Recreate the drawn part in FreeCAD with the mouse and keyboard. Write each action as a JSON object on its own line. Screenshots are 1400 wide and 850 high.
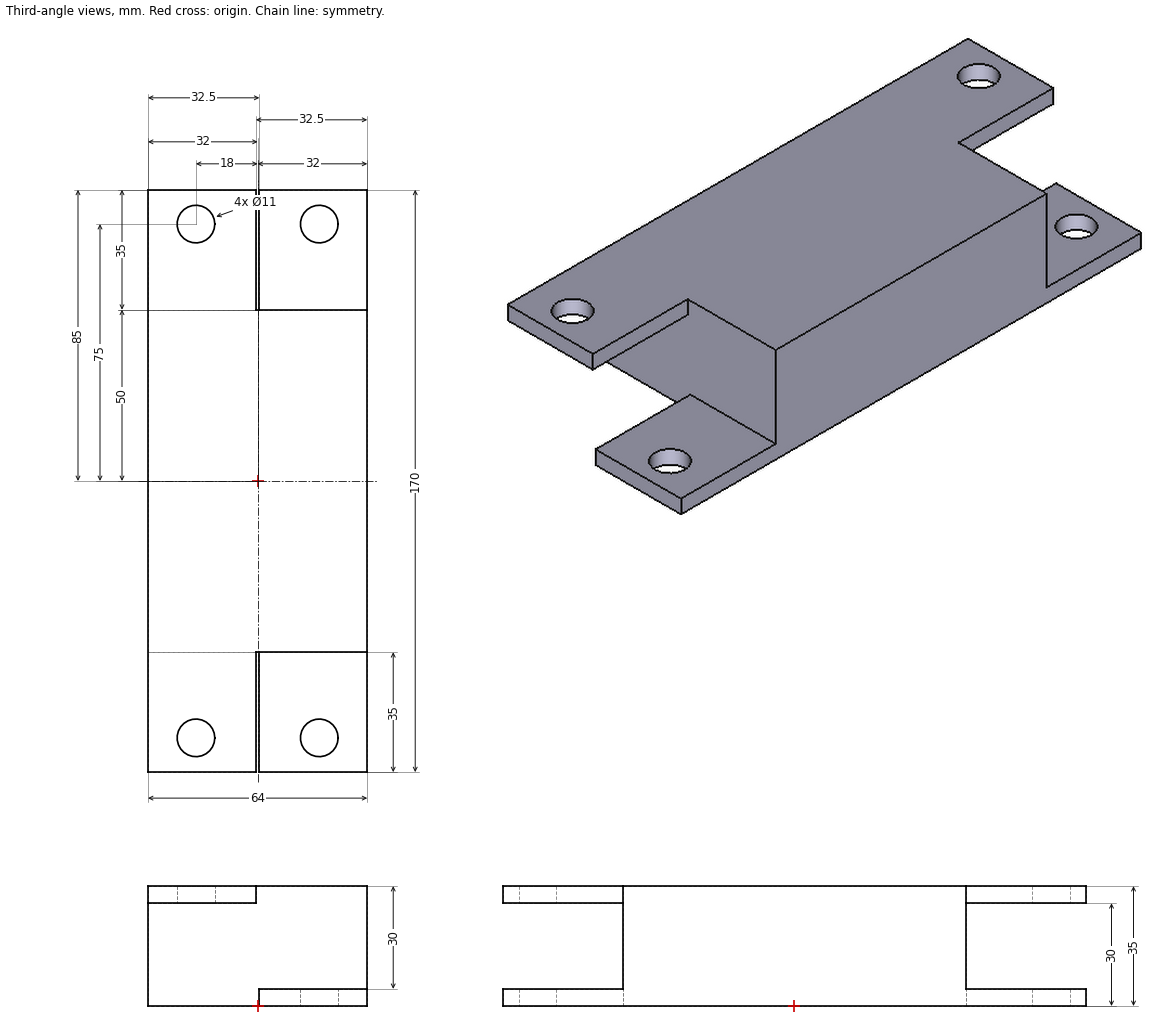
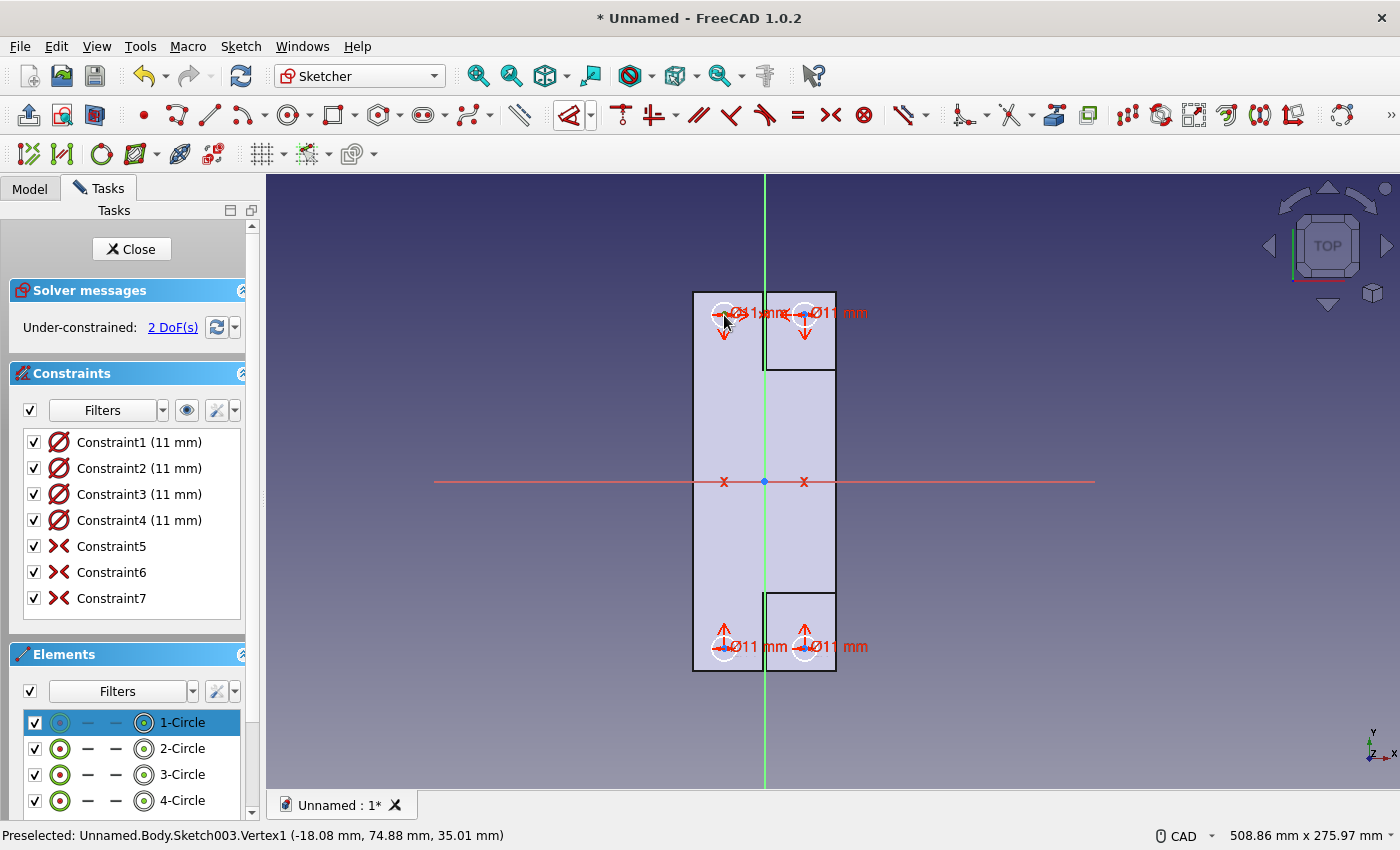
{"action": "left_click", "coordinate": [590, 116]}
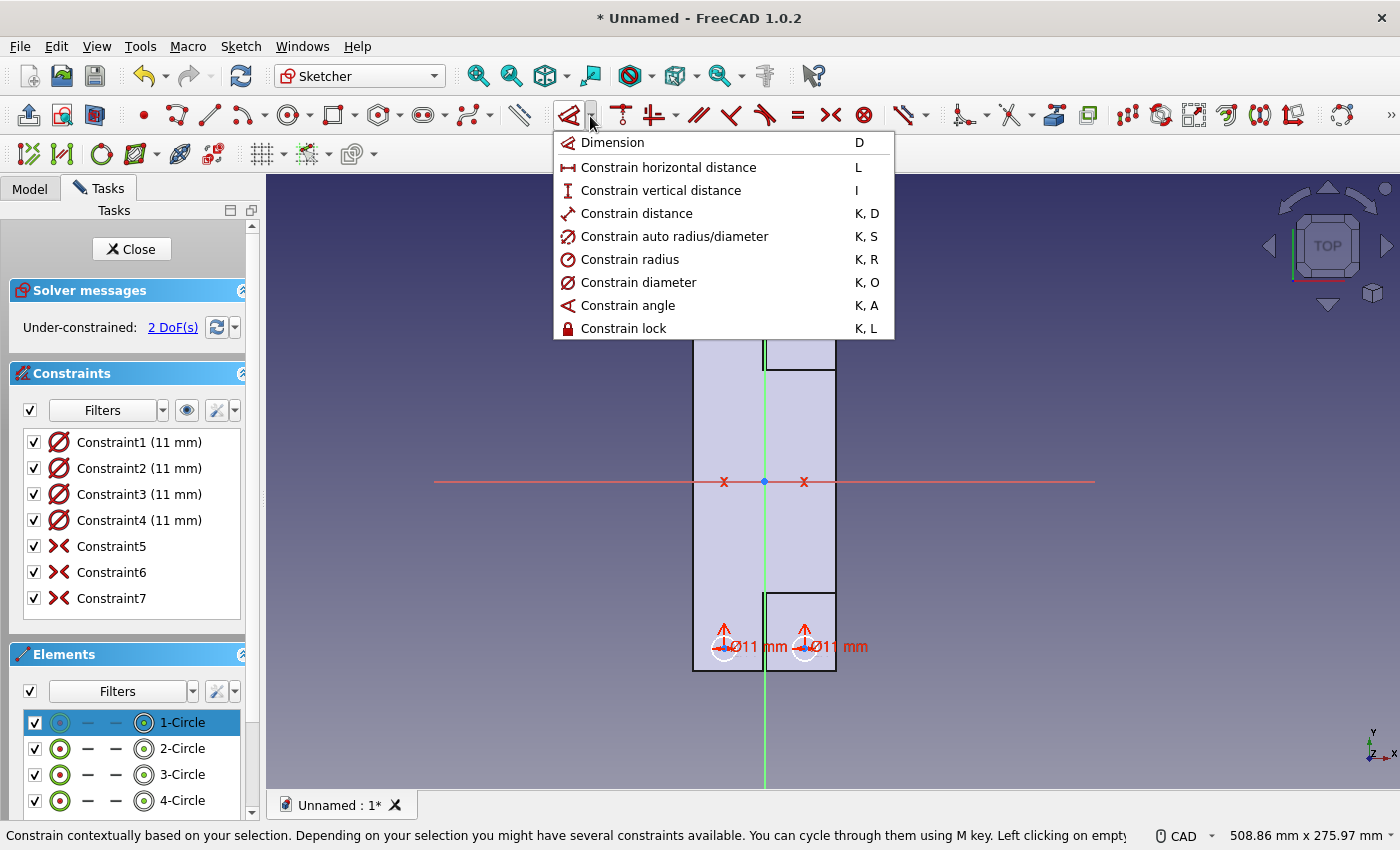
{"action": "left_click", "coordinate": [724, 168]}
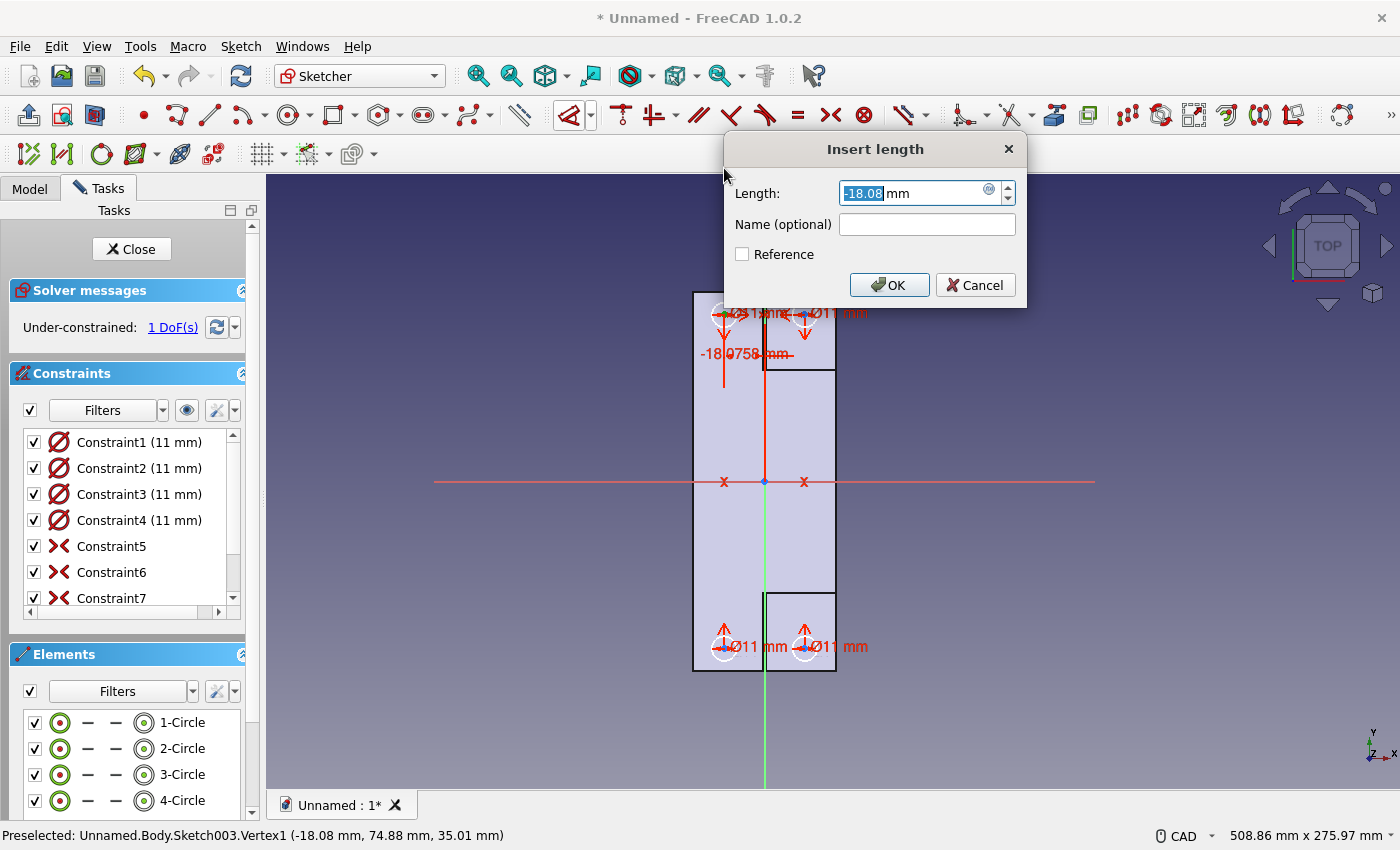
{"action": "type", "text": "-18"}
{"action": "key", "text": "Return"}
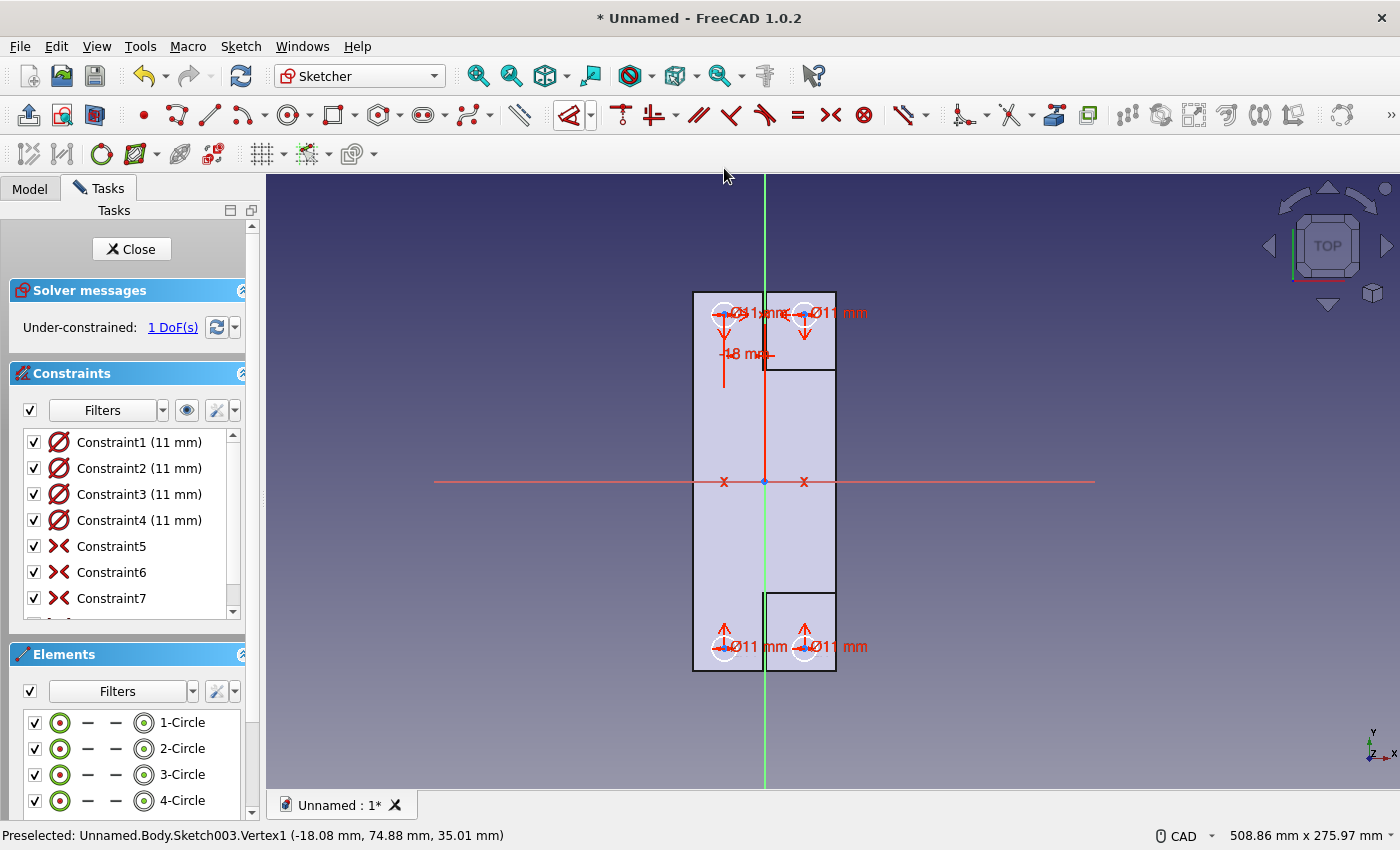
{"action": "left_click", "coordinate": [724, 315]}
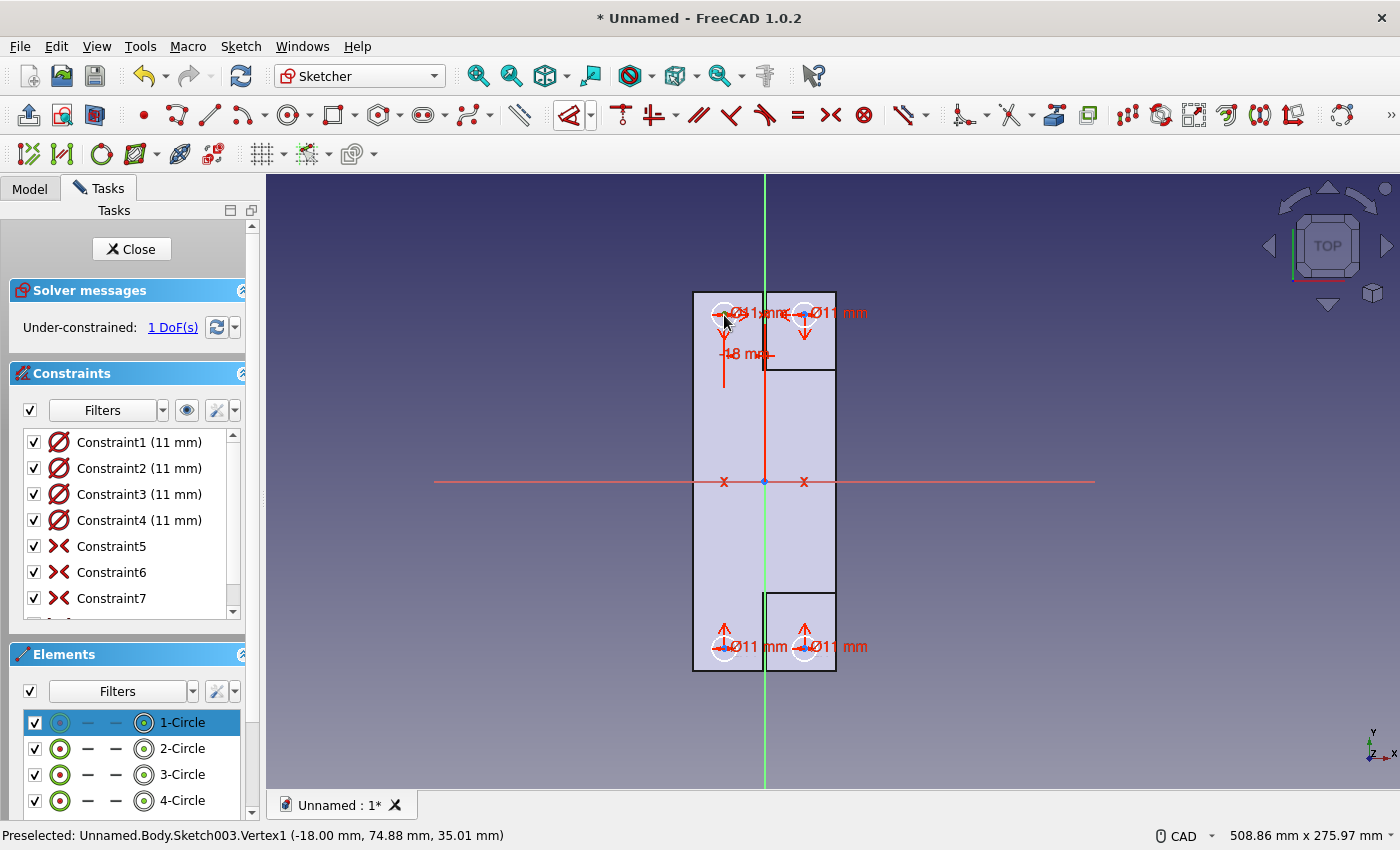
{"action": "key", "text": "i"}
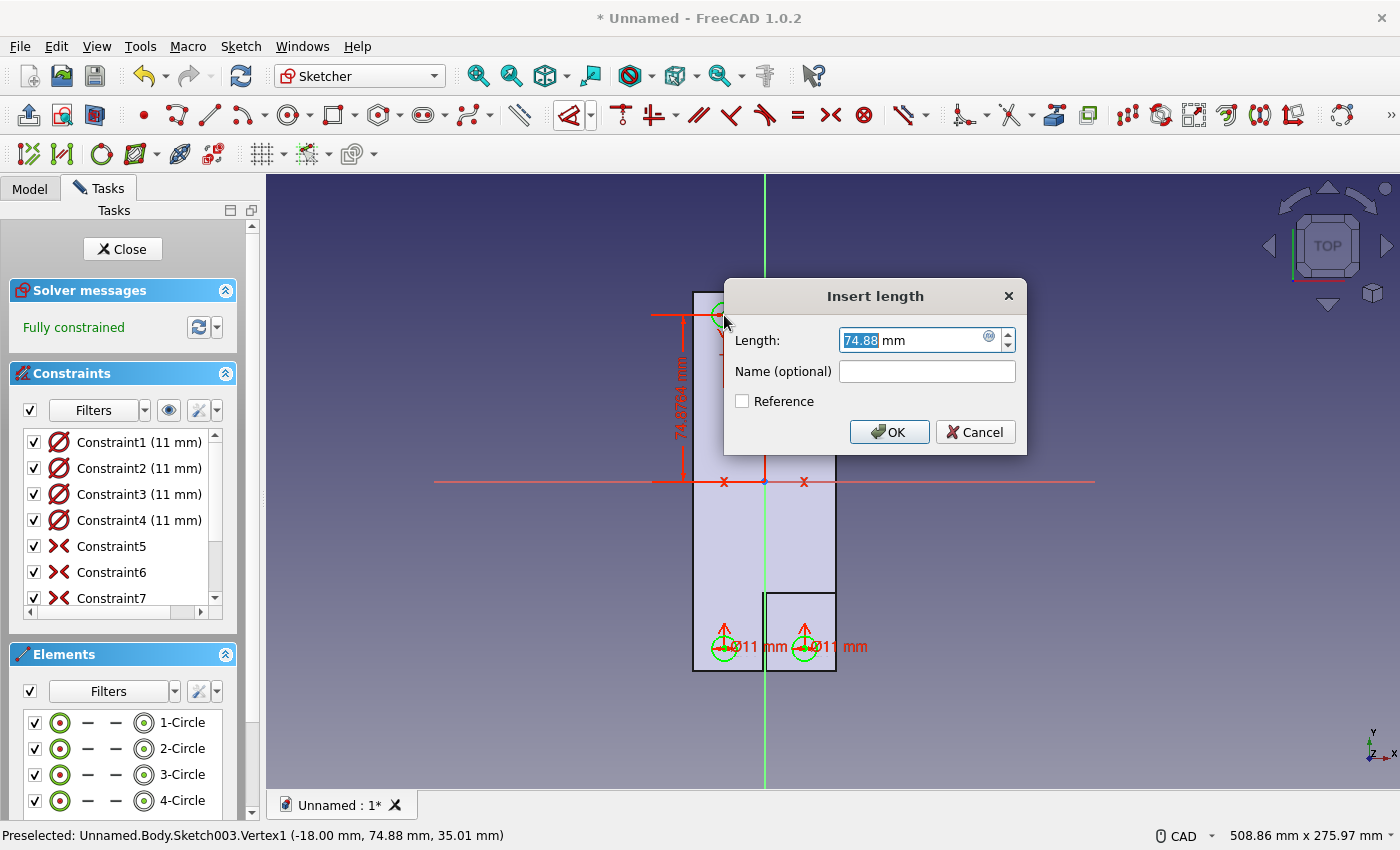
{"action": "type", "text": "75"}
{"action": "key", "text": "Return"}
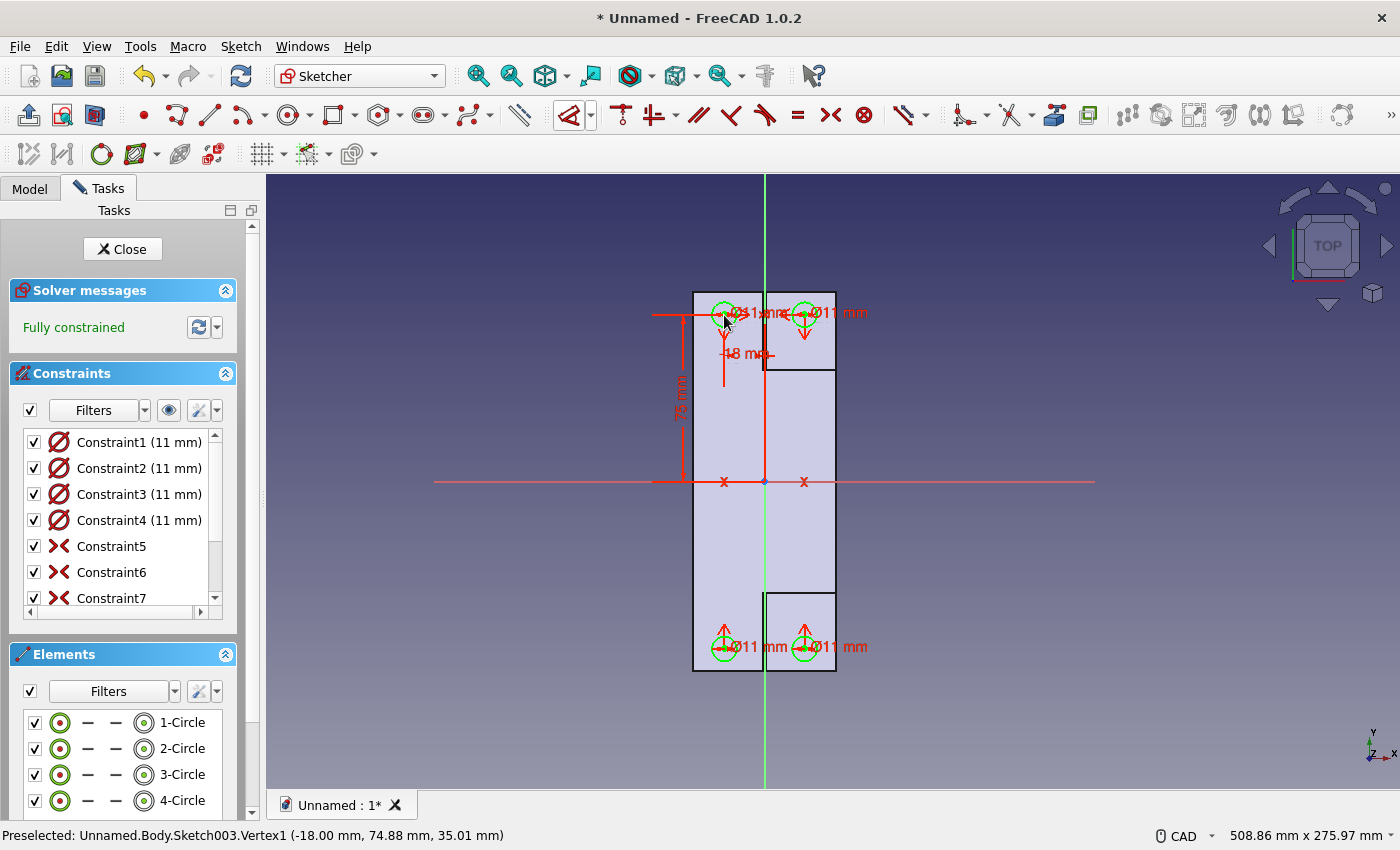
{"action": "left_click", "coordinate": [123, 249]}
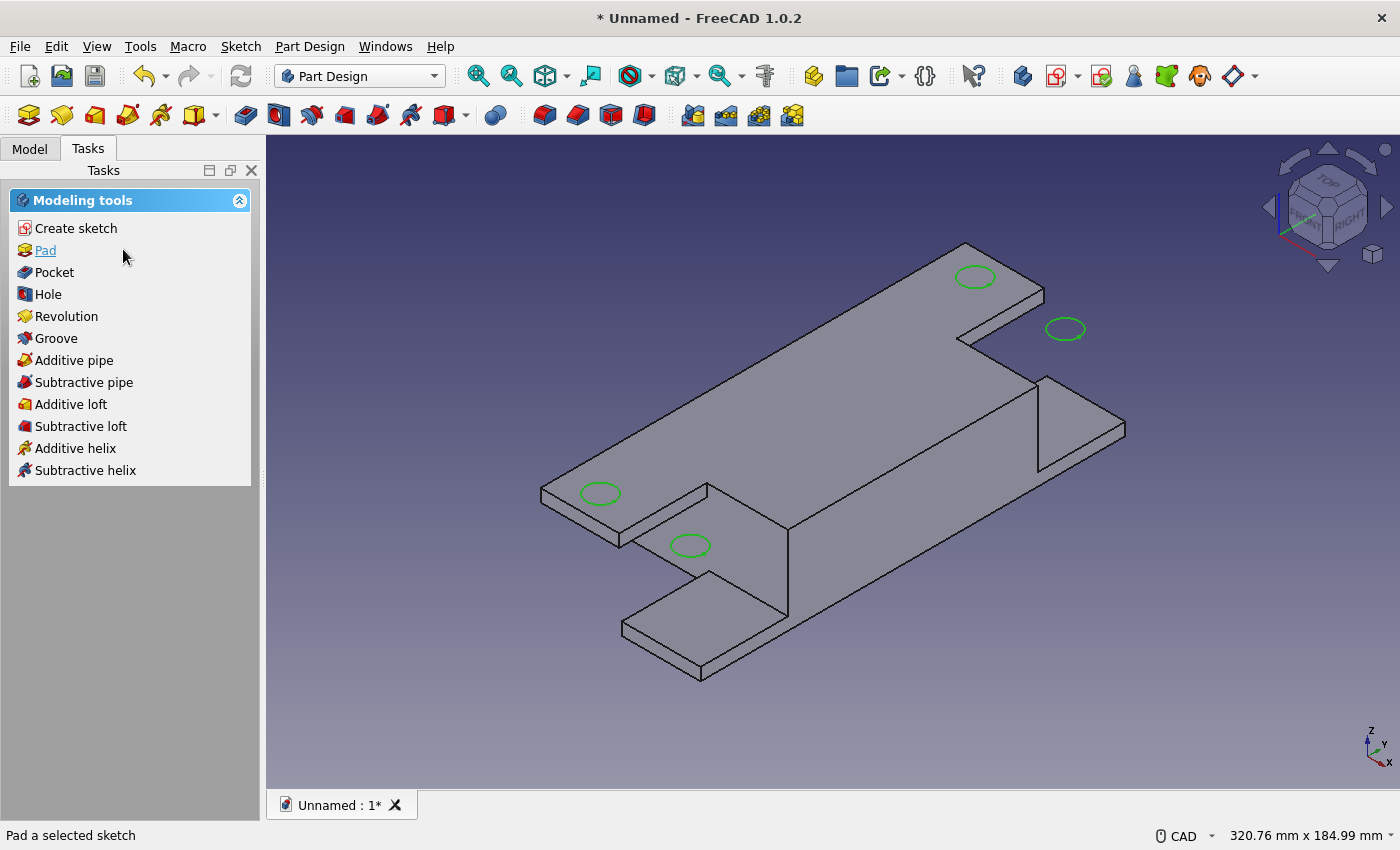
{"action": "left_click", "coordinate": [246, 116]}